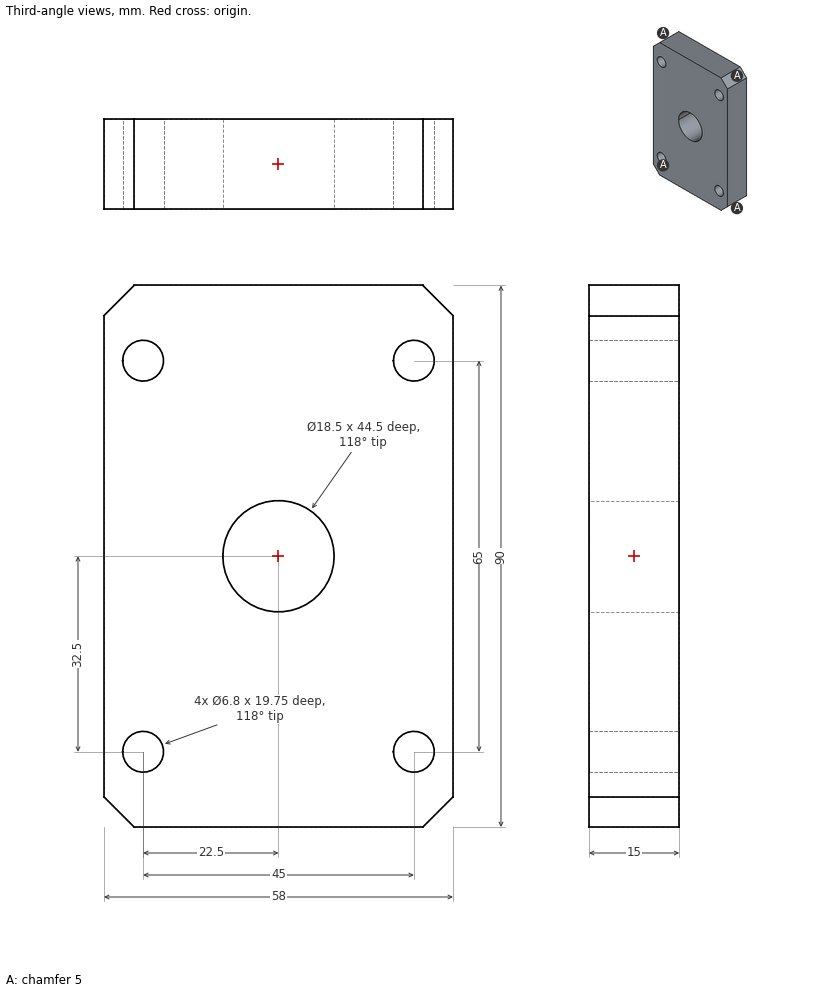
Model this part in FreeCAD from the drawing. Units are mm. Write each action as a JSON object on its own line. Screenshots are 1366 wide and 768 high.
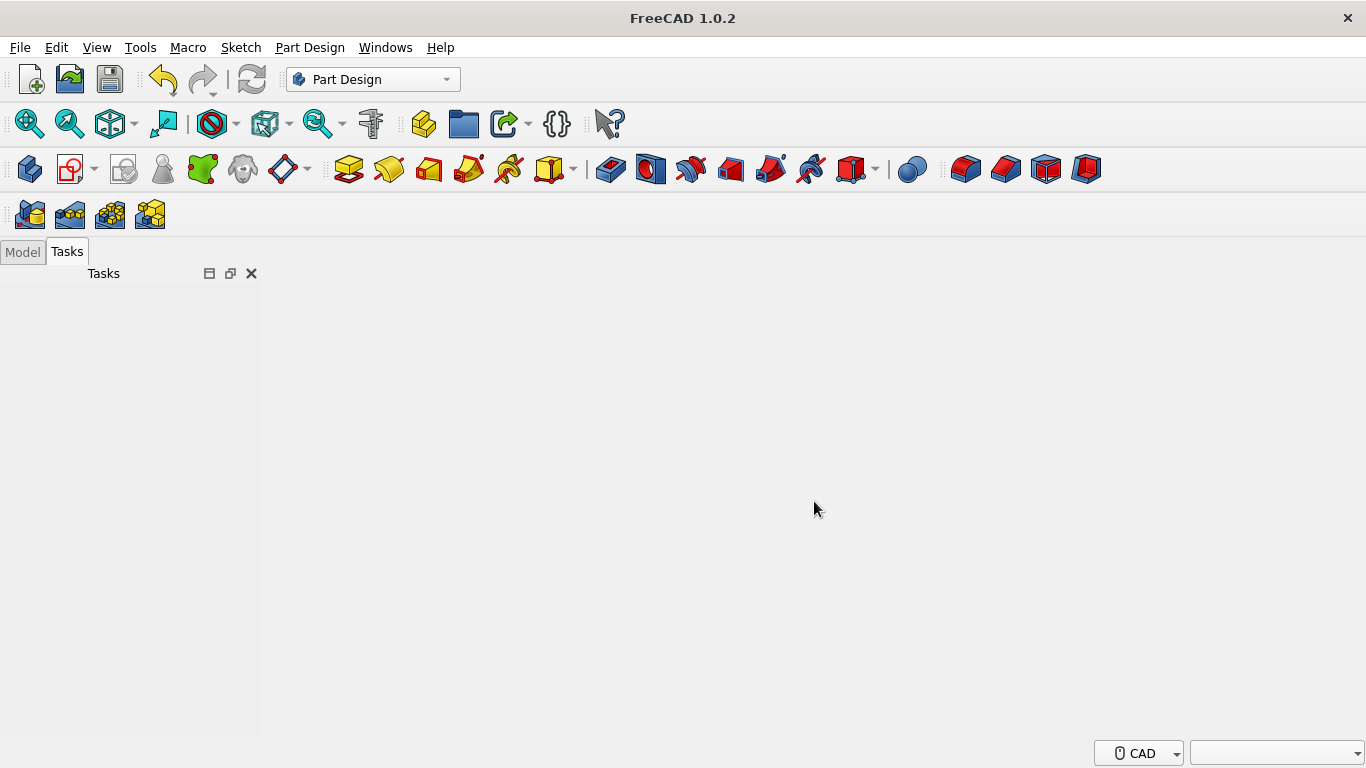
{"action": "key", "text": "ctrl+n"}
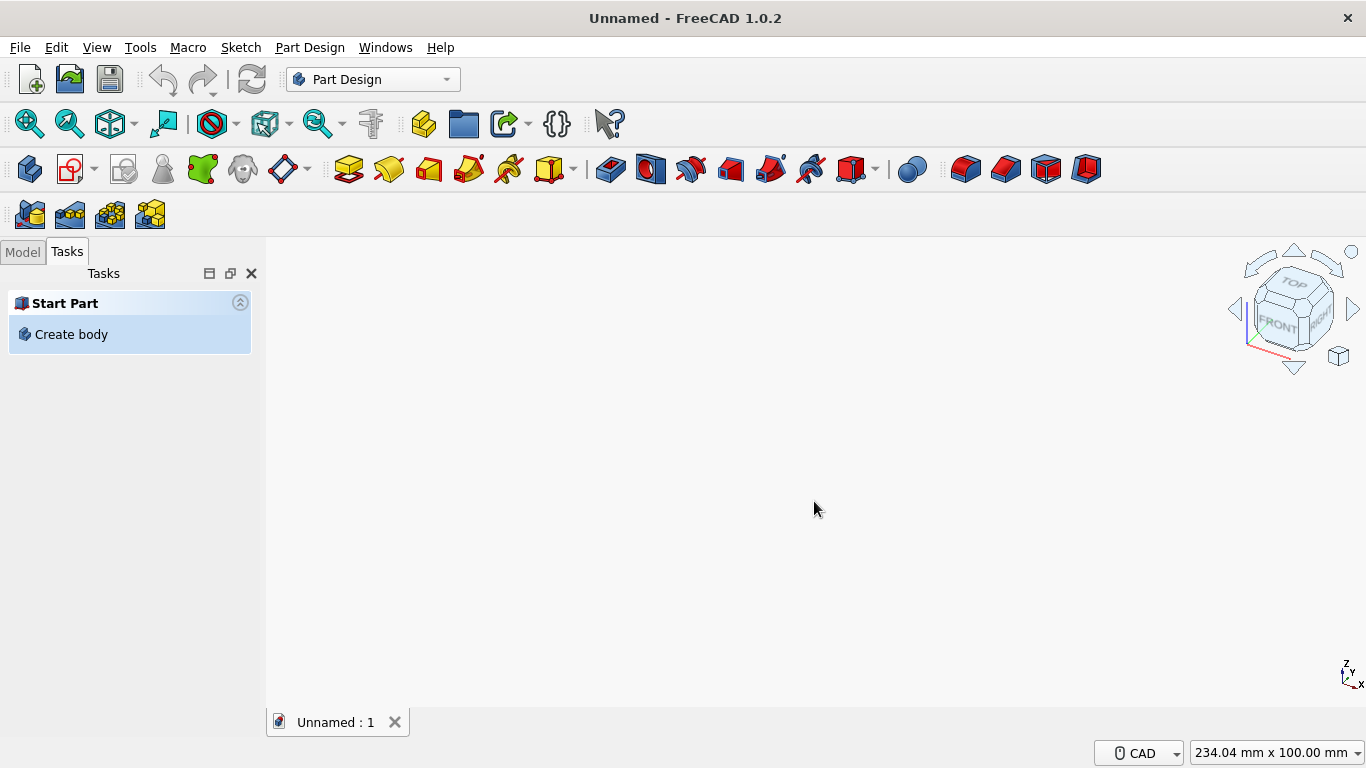
{"action": "left_click", "coordinate": [70, 170]}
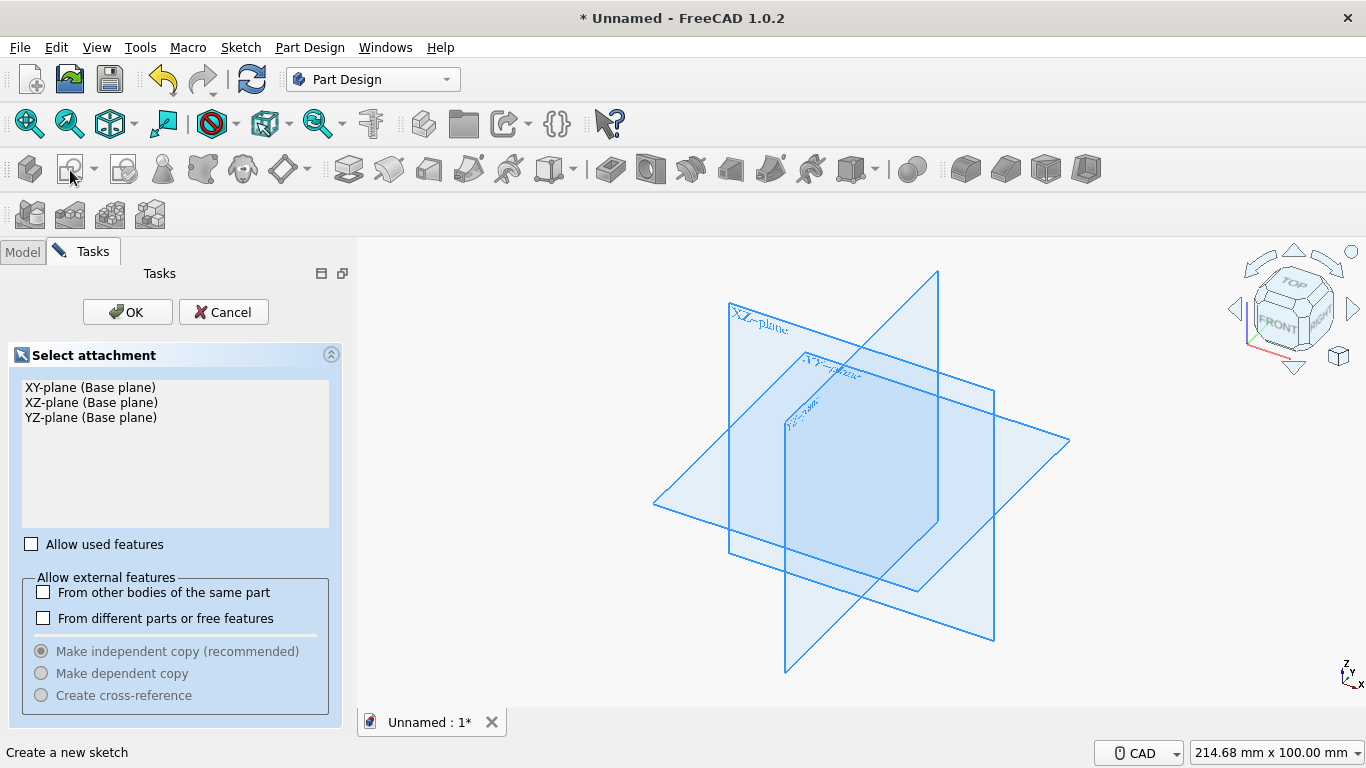
{"action": "left_click", "coordinate": [82, 402]}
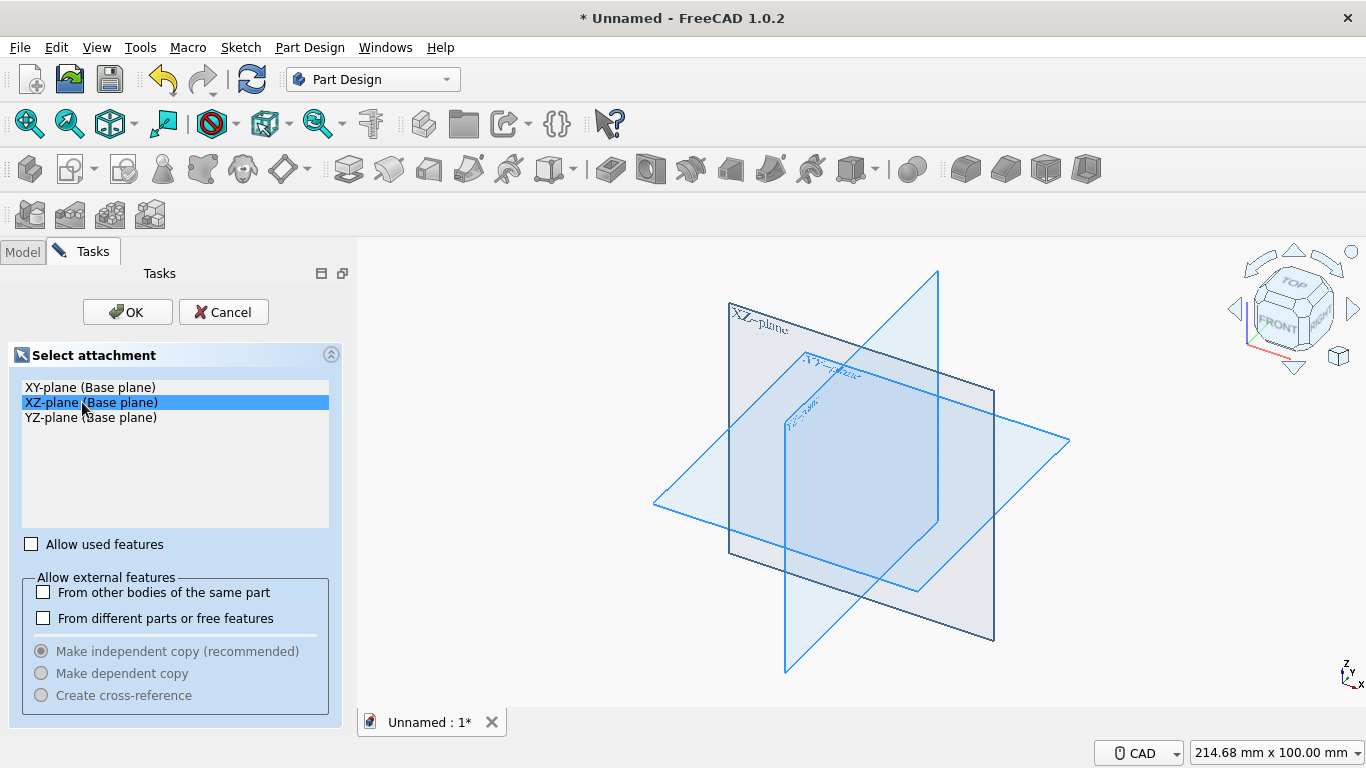
{"action": "left_click", "coordinate": [128, 312]}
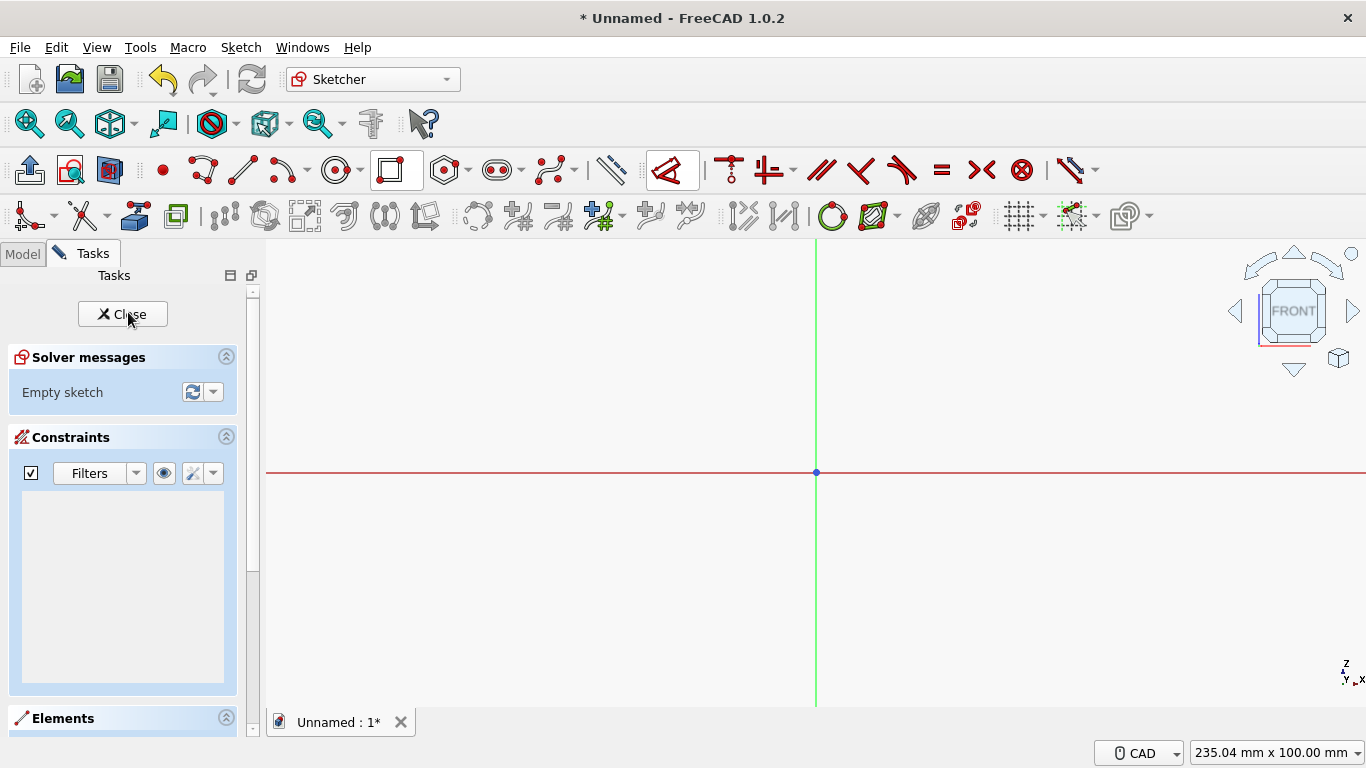
{"action": "scroll", "coordinate": [608, 473], "scroll_direction": "down", "scroll_amount": 2}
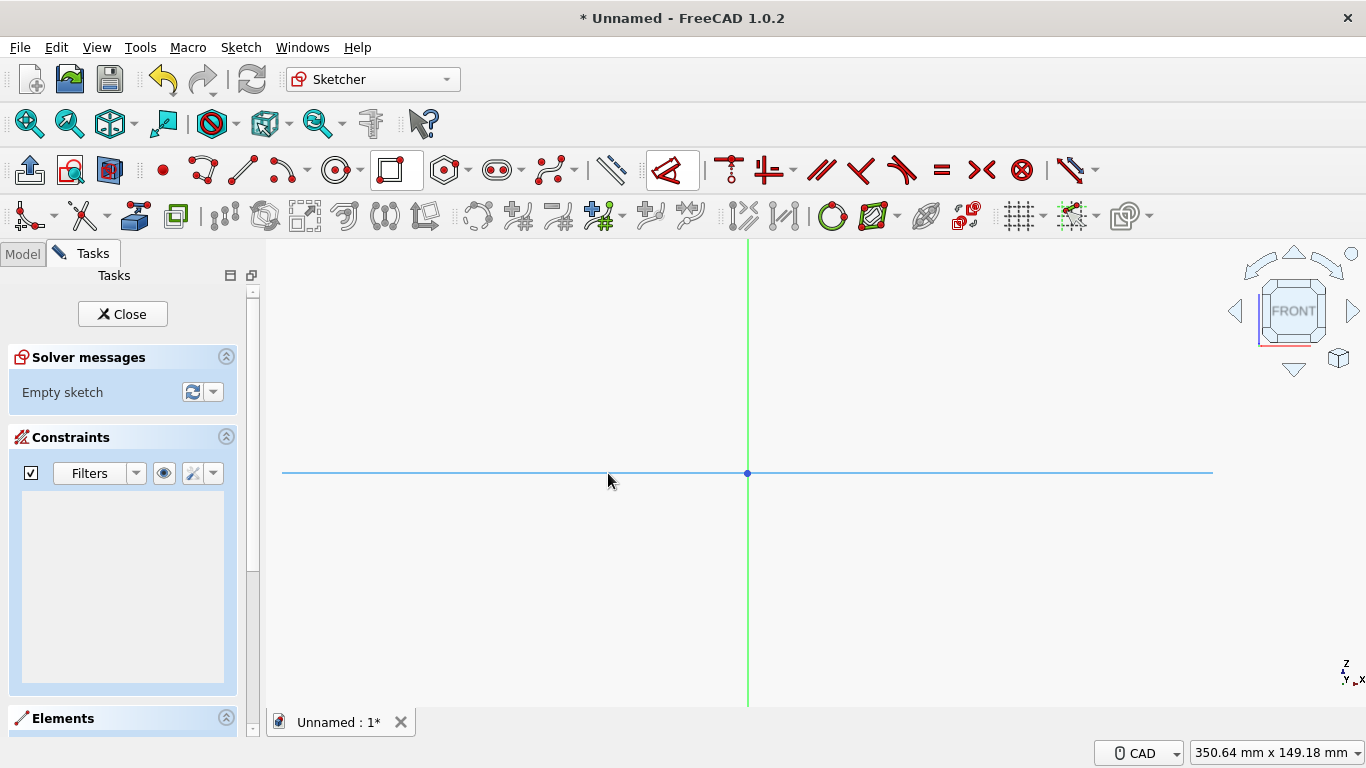
{"action": "key", "text": "g v"}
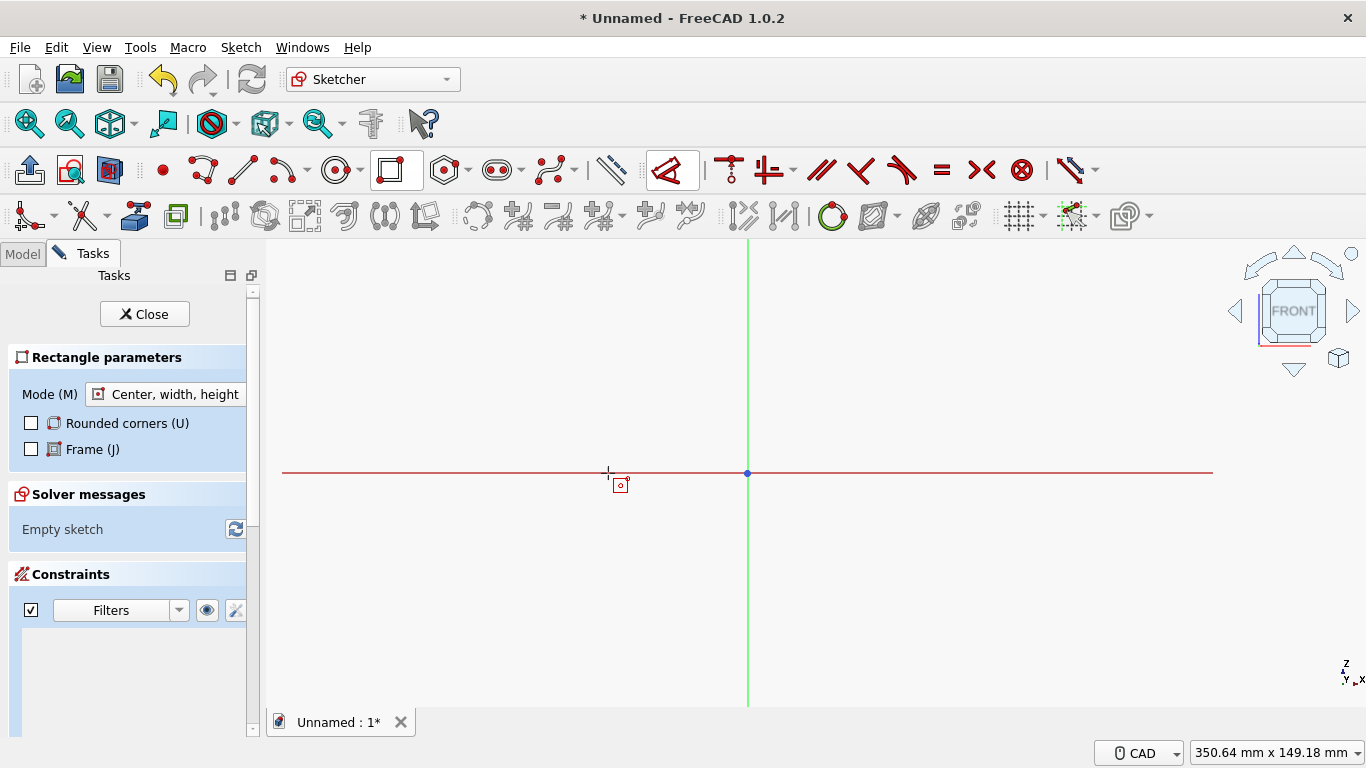
{"action": "left_click", "coordinate": [748, 473]}
{"action": "left_click", "coordinate": [839, 332]}
{"action": "key", "text": "Escape"}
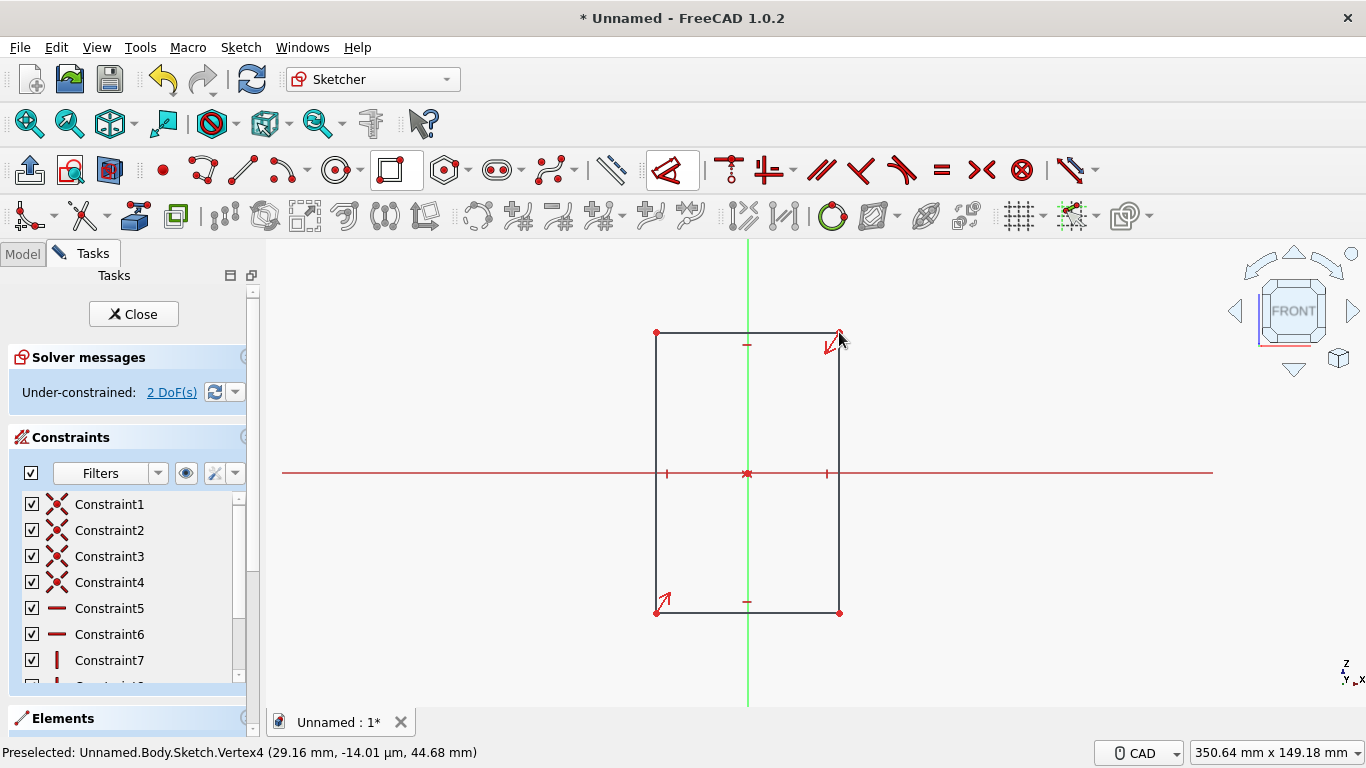
{"action": "left_click", "coordinate": [666, 170]}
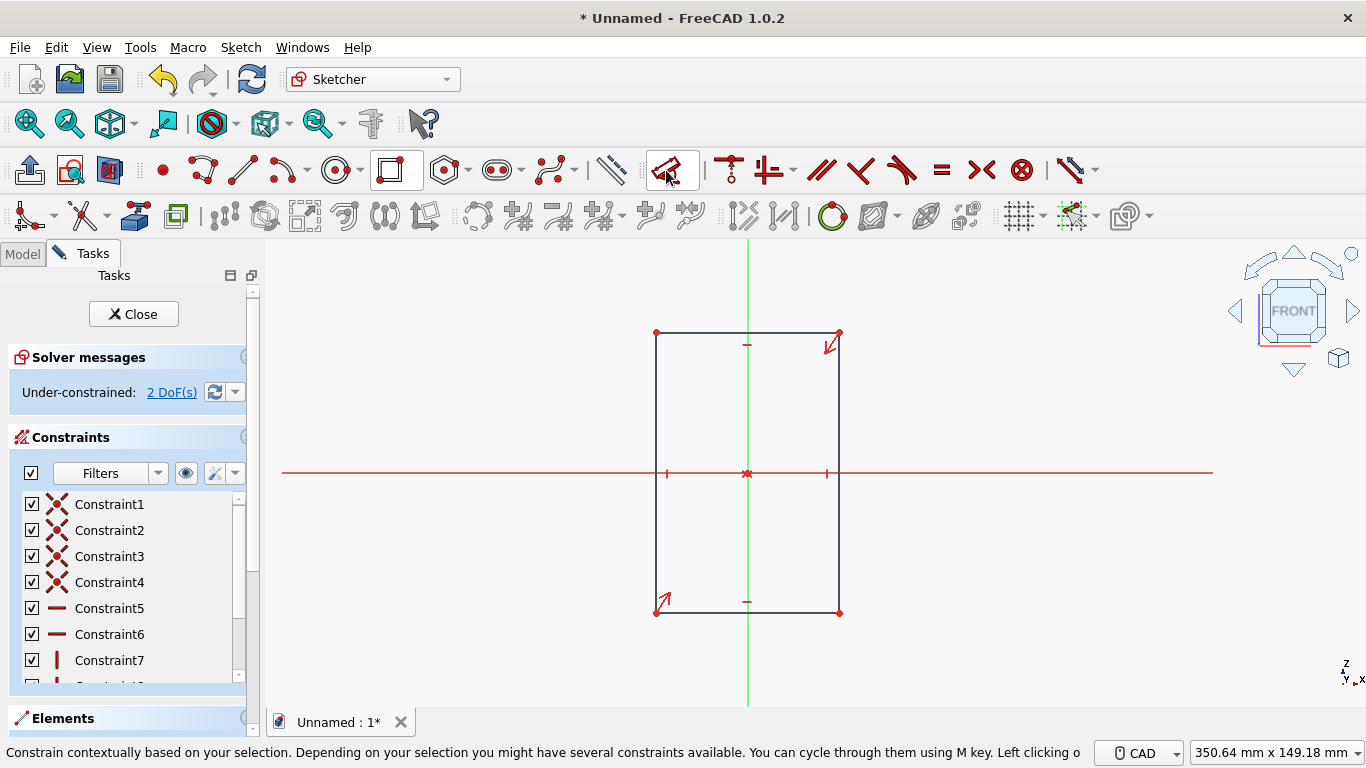
{"action": "left_click", "coordinate": [711, 613]}
{"action": "left_click", "coordinate": [705, 647]}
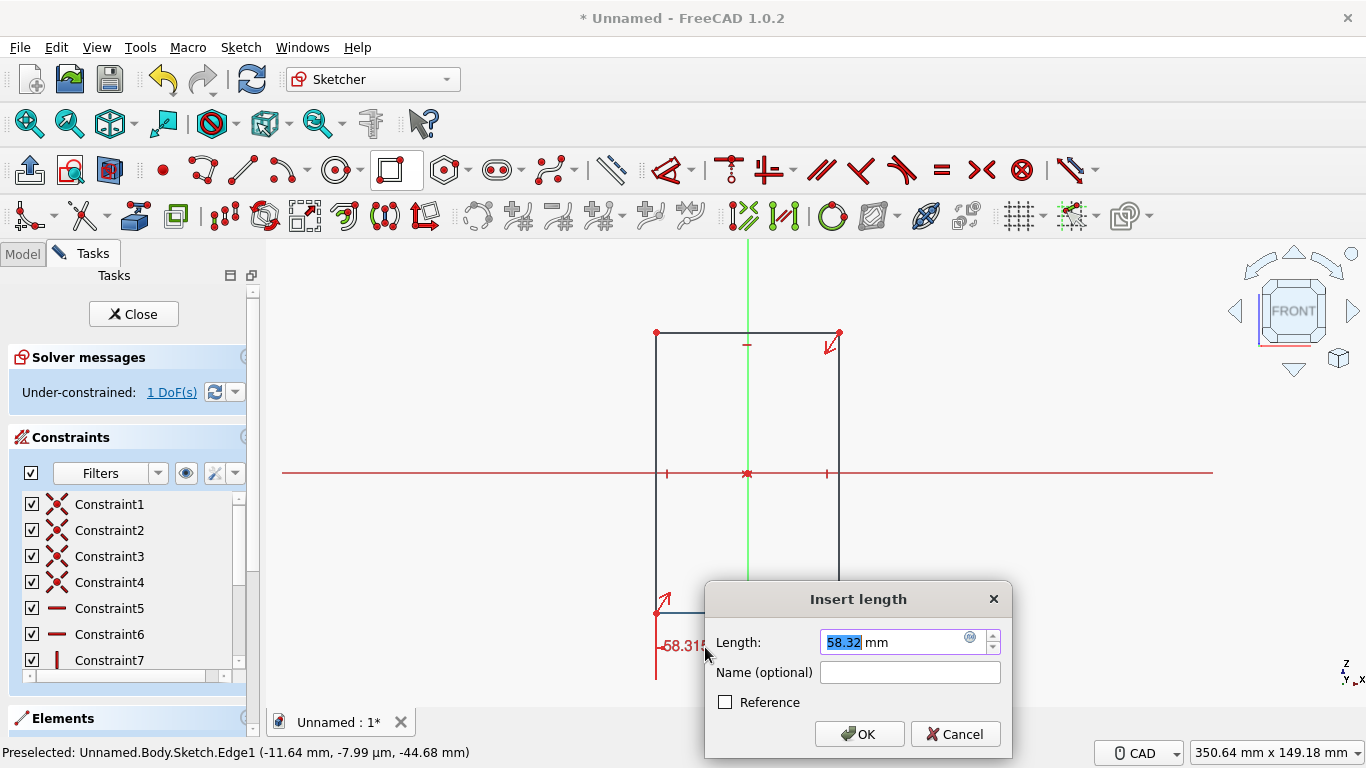
{"action": "type", "text": "58"}
{"action": "key", "text": "Return"}